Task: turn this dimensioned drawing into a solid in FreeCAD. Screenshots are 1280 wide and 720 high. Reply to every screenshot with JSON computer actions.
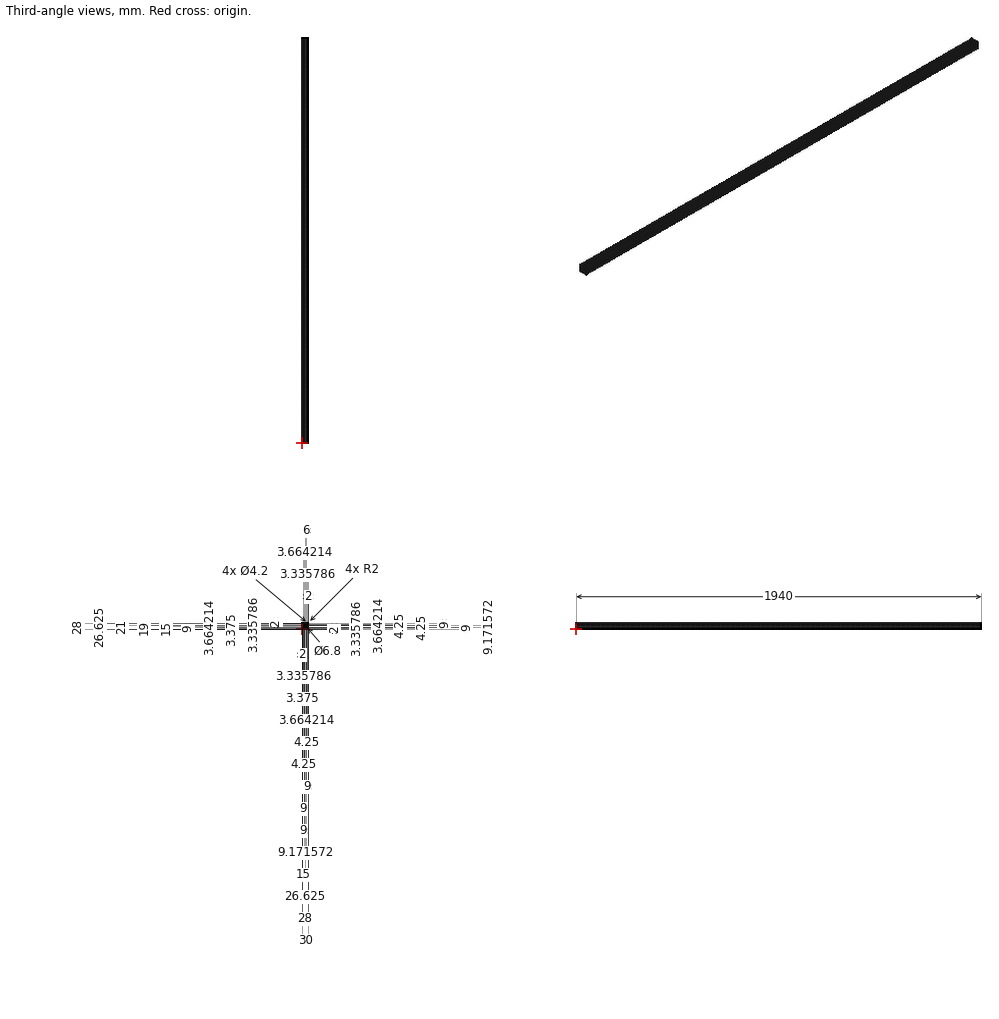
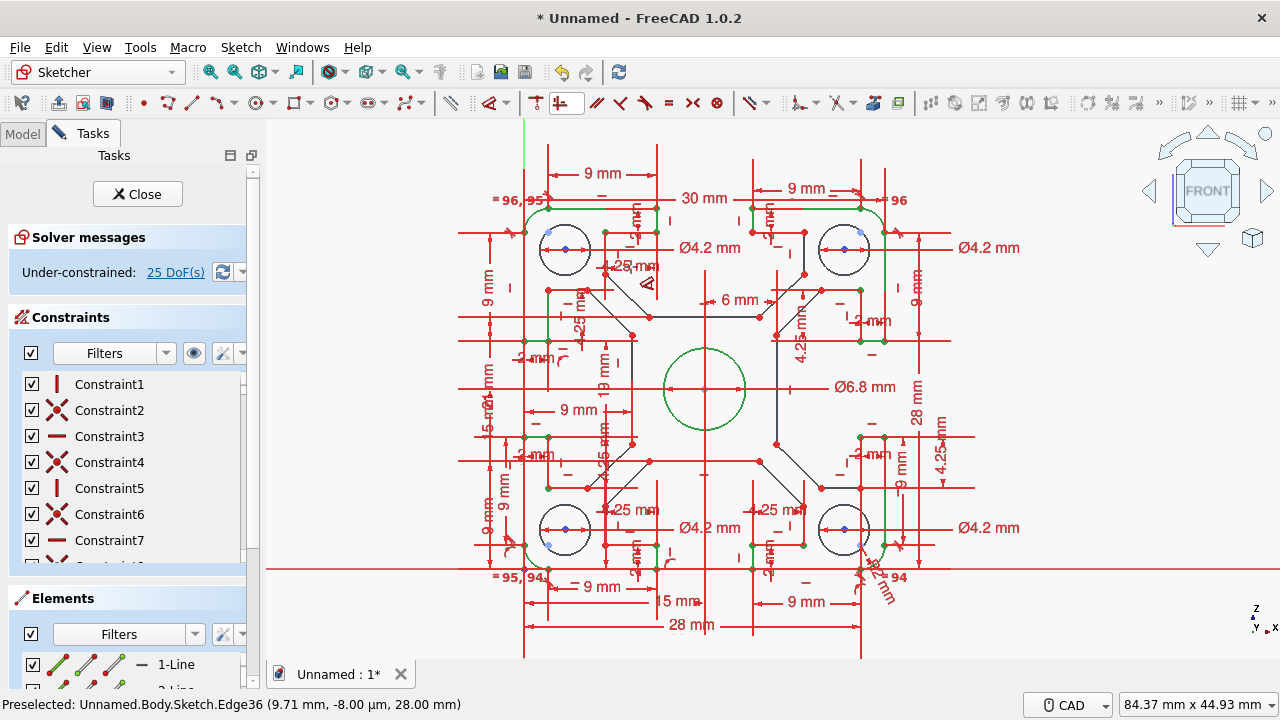
{"action": "left_click", "coordinate": [789, 233]}
{"action": "left_click", "coordinate": [778, 267]}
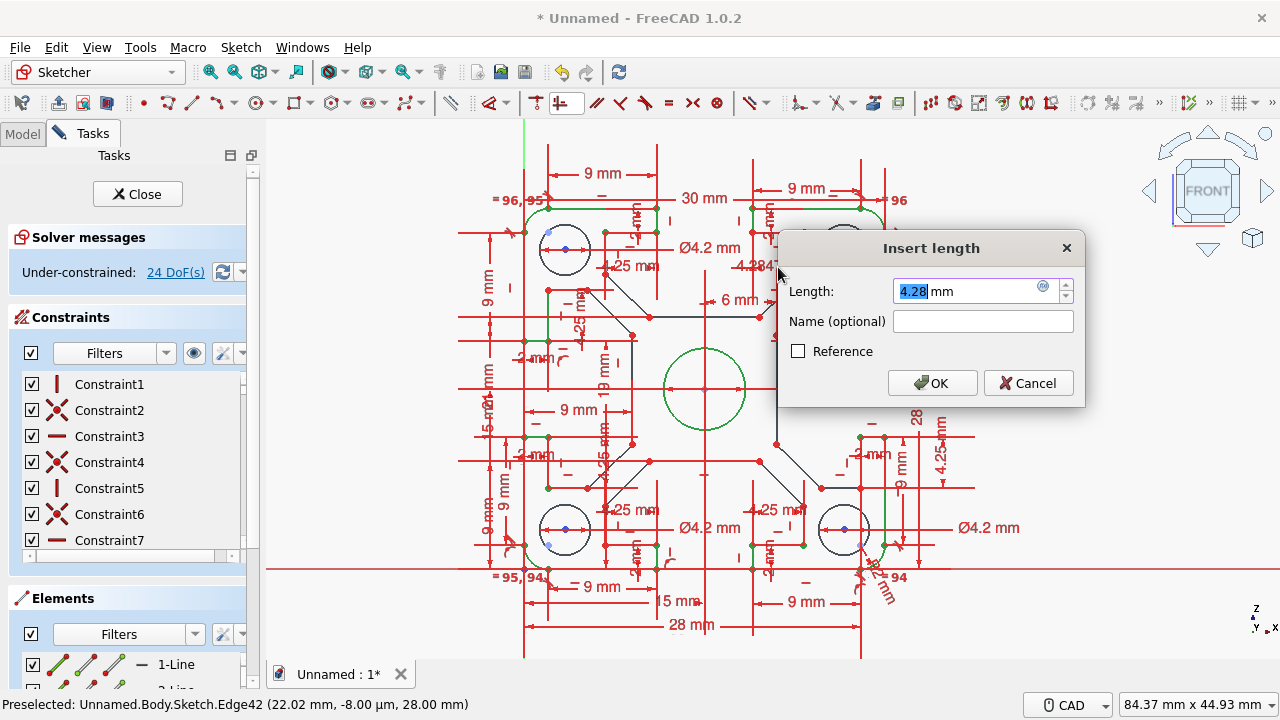
{"action": "type", "text": "4.25"}
{"action": "key", "text": "Return"}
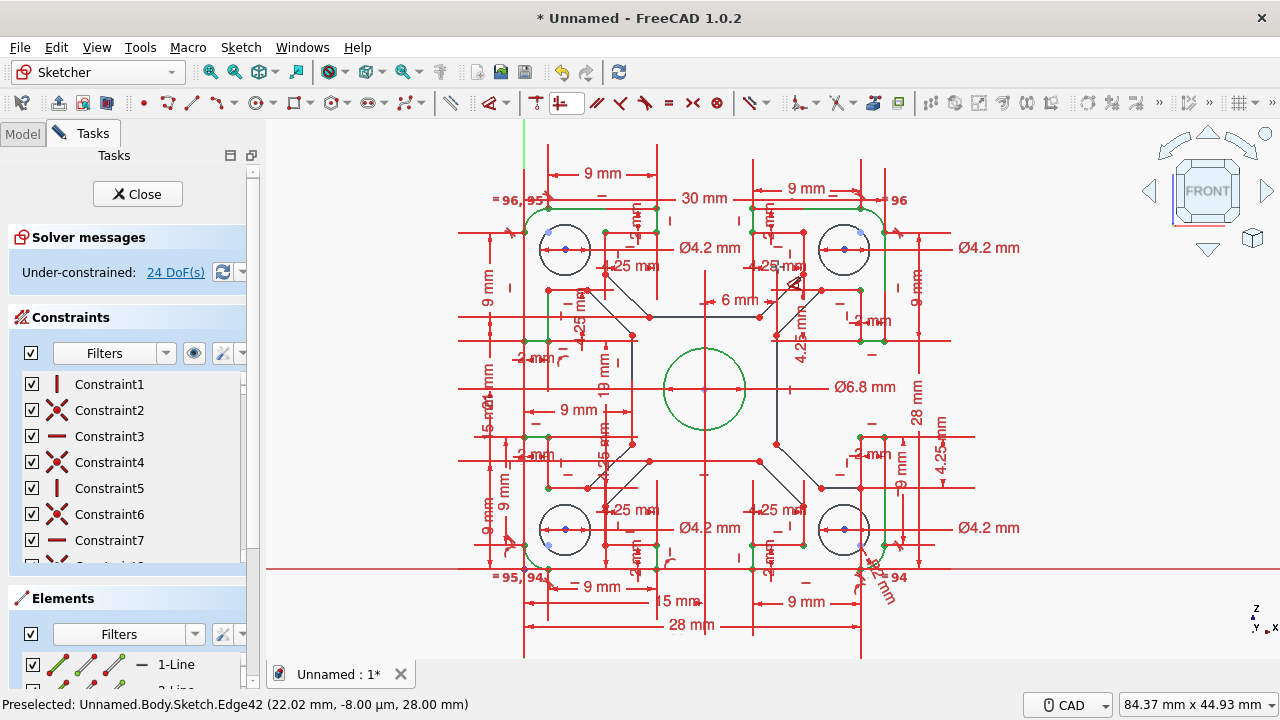
{"action": "left_click", "coordinate": [565, 250]}
{"action": "left_click", "coordinate": [545, 627]}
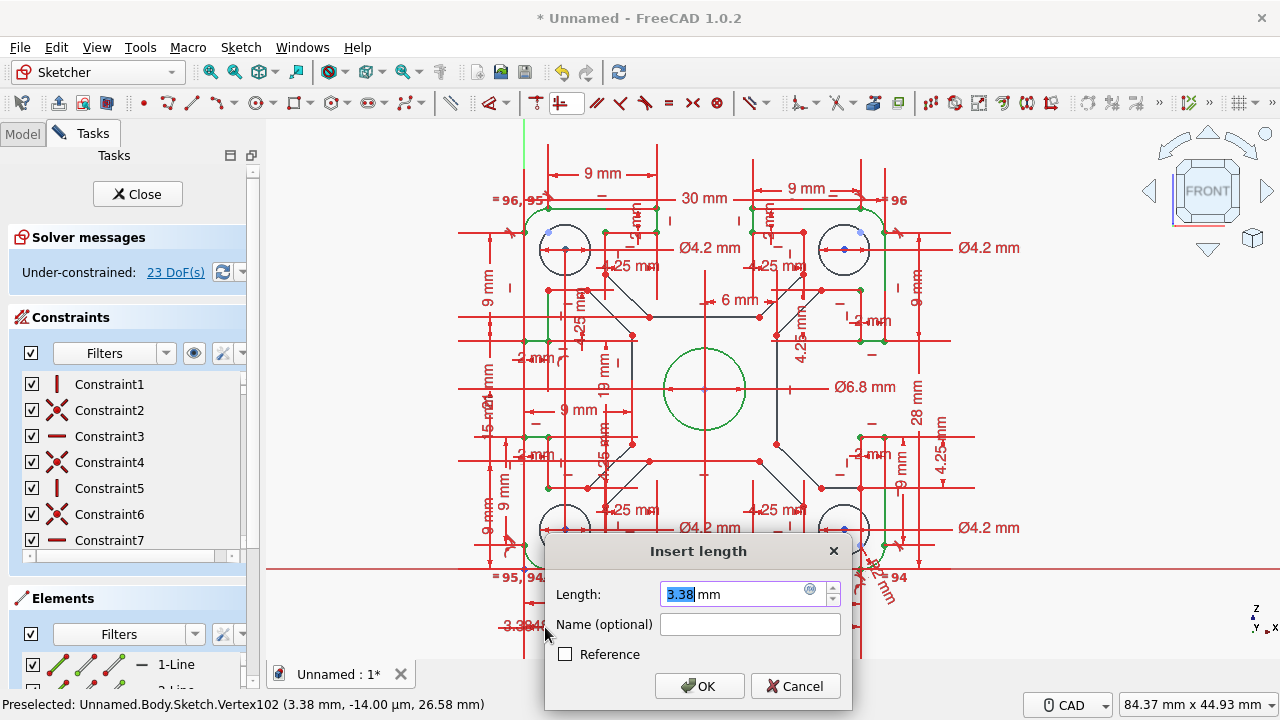
{"action": "type", "text": "3.375"}
{"action": "key", "text": "Return"}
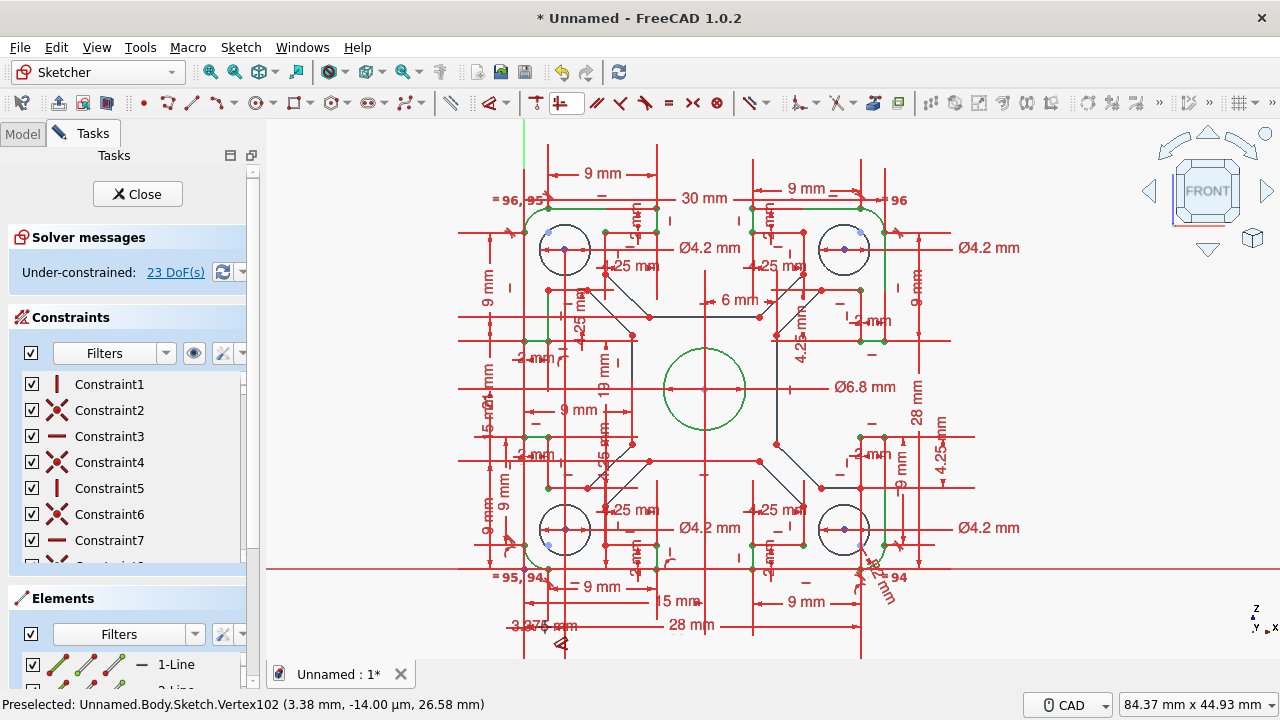
{"action": "left_click", "coordinate": [844, 530]}
{"action": "left_click", "coordinate": [490, 550]}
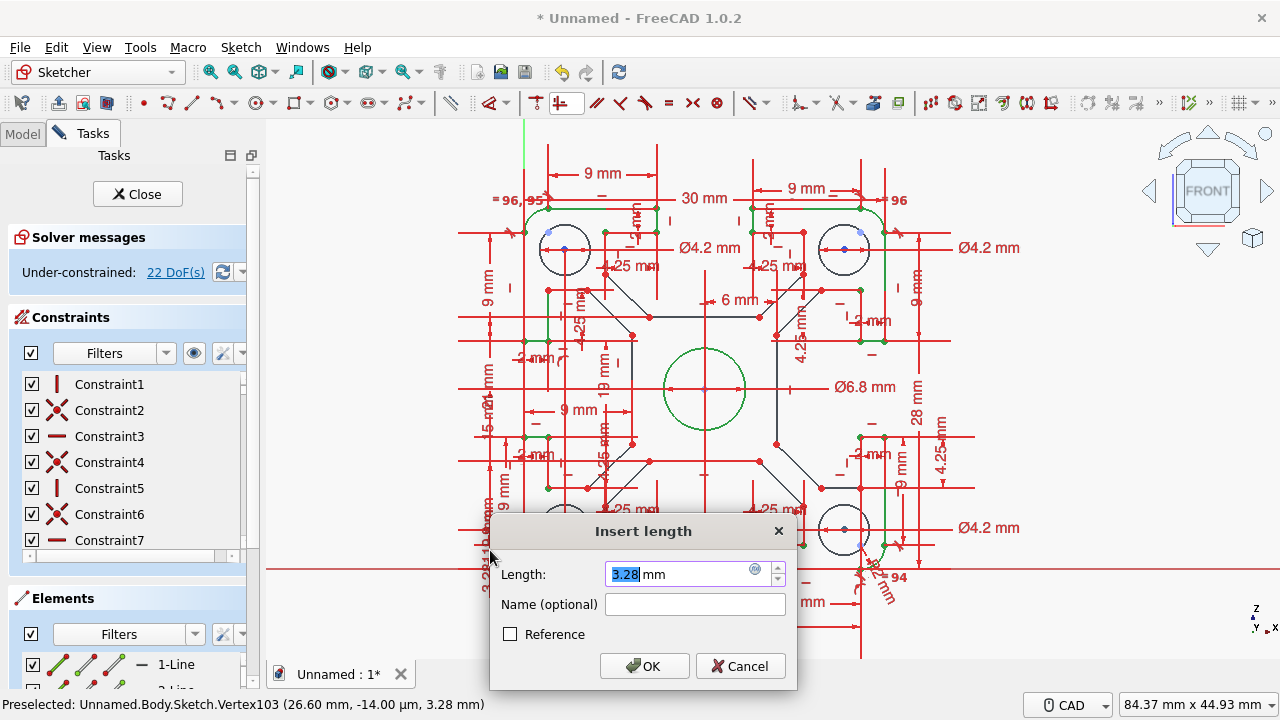
{"action": "type", "text": "3.375"}
{"action": "key", "text": "Return"}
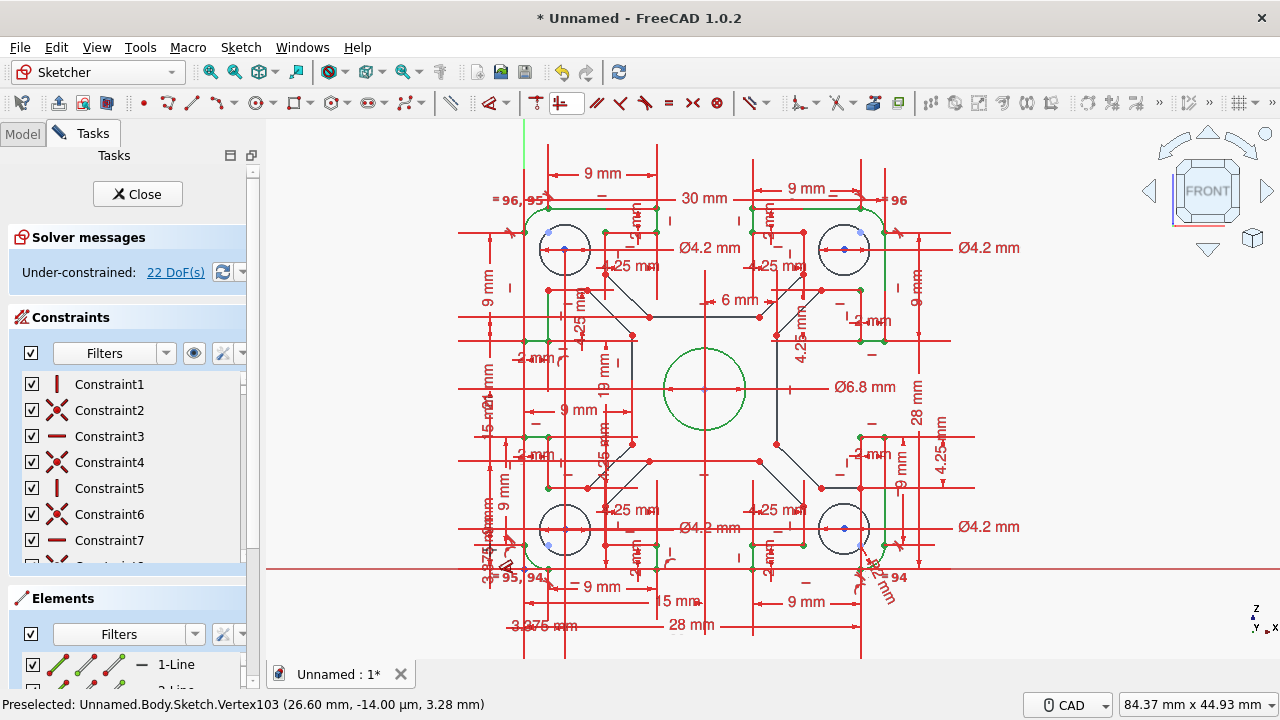
{"action": "left_click", "coordinate": [565, 530]}
{"action": "left_click", "coordinate": [545, 603]}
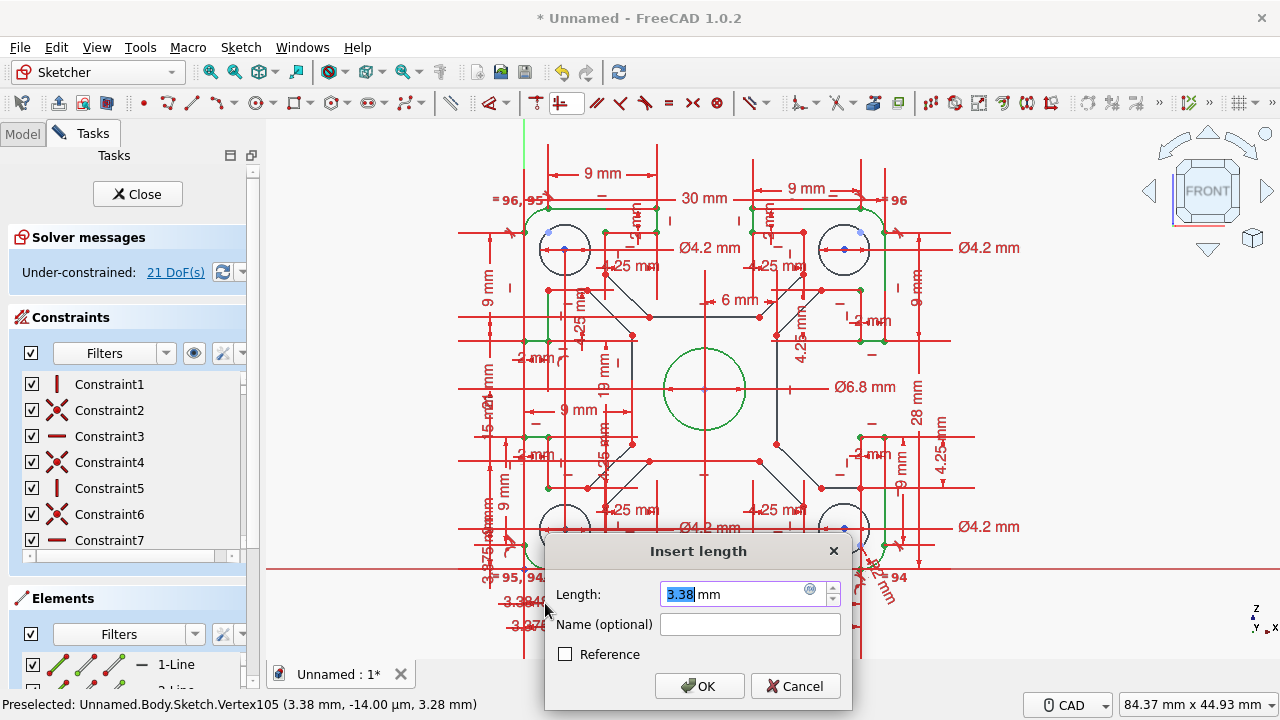
{"action": "type", "text": "3.375"}
{"action": "key", "text": "Return"}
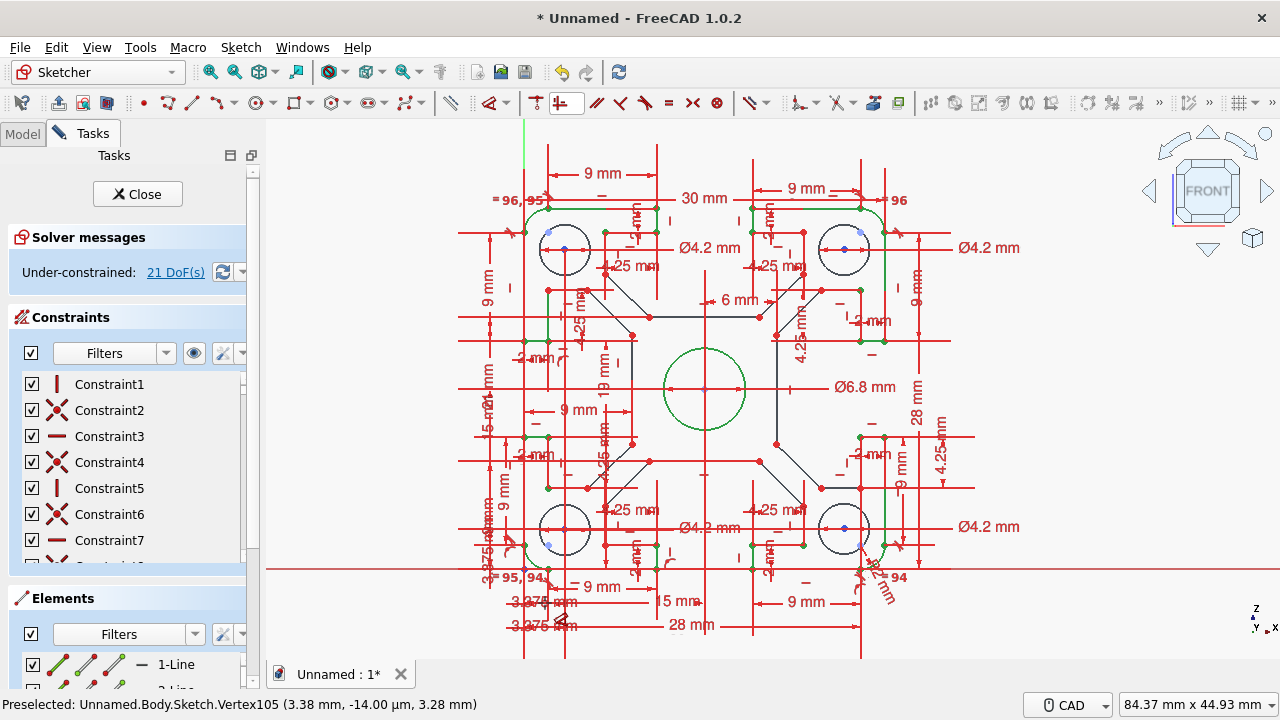
{"action": "left_click", "coordinate": [565, 530]}
{"action": "left_click", "coordinate": [418, 550]}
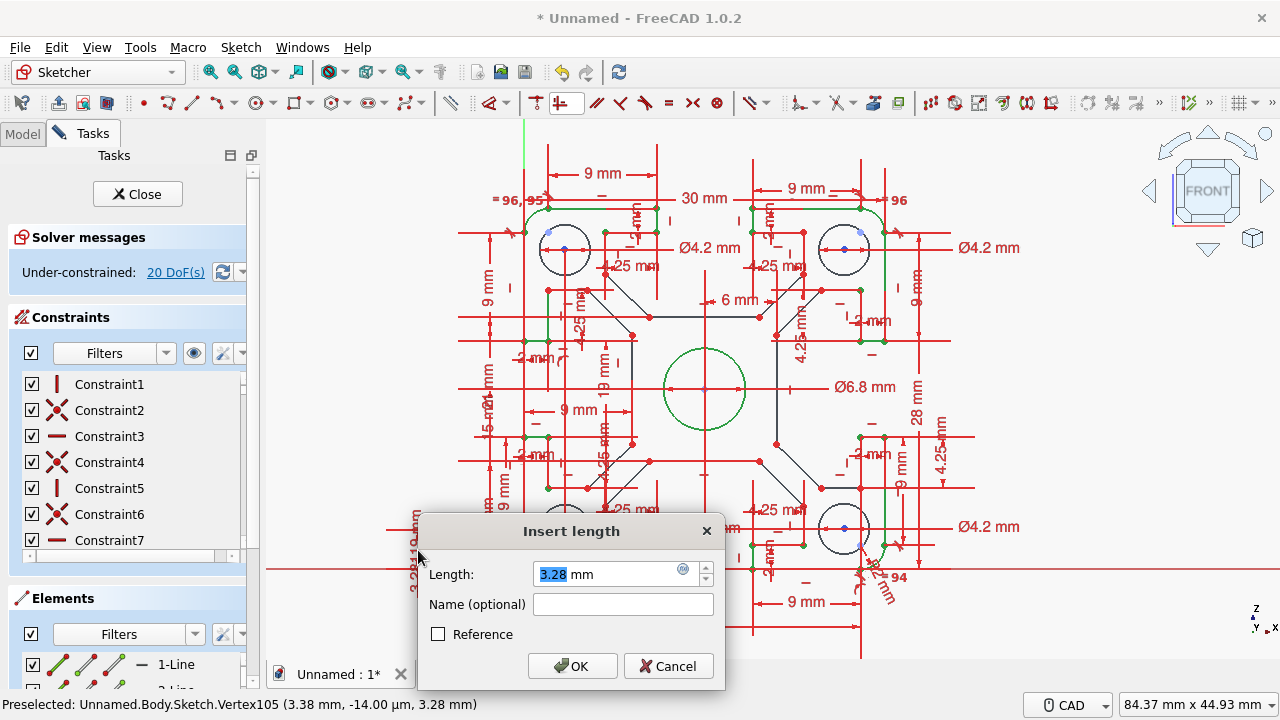
{"action": "type", "text": "3.375"}
{"action": "key", "text": "Return"}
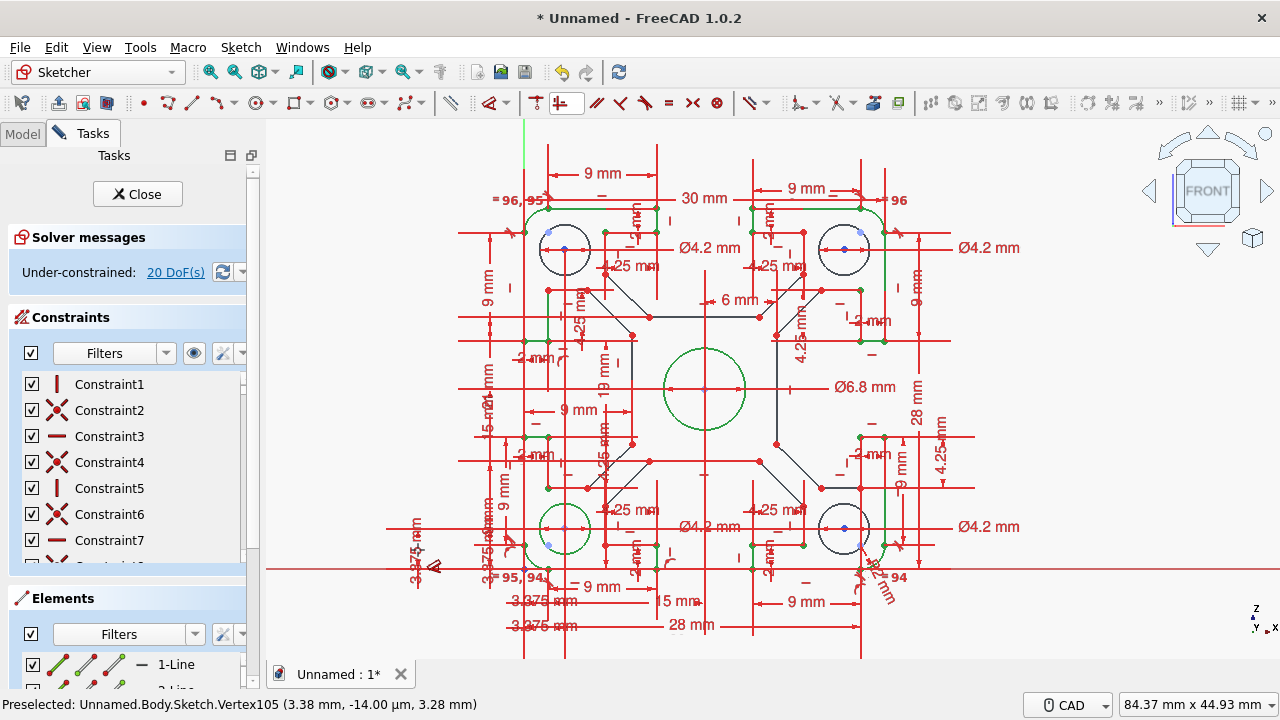
{"action": "left_click", "coordinate": [844, 250]}
{"action": "left_click", "coordinate": [796, 627]}